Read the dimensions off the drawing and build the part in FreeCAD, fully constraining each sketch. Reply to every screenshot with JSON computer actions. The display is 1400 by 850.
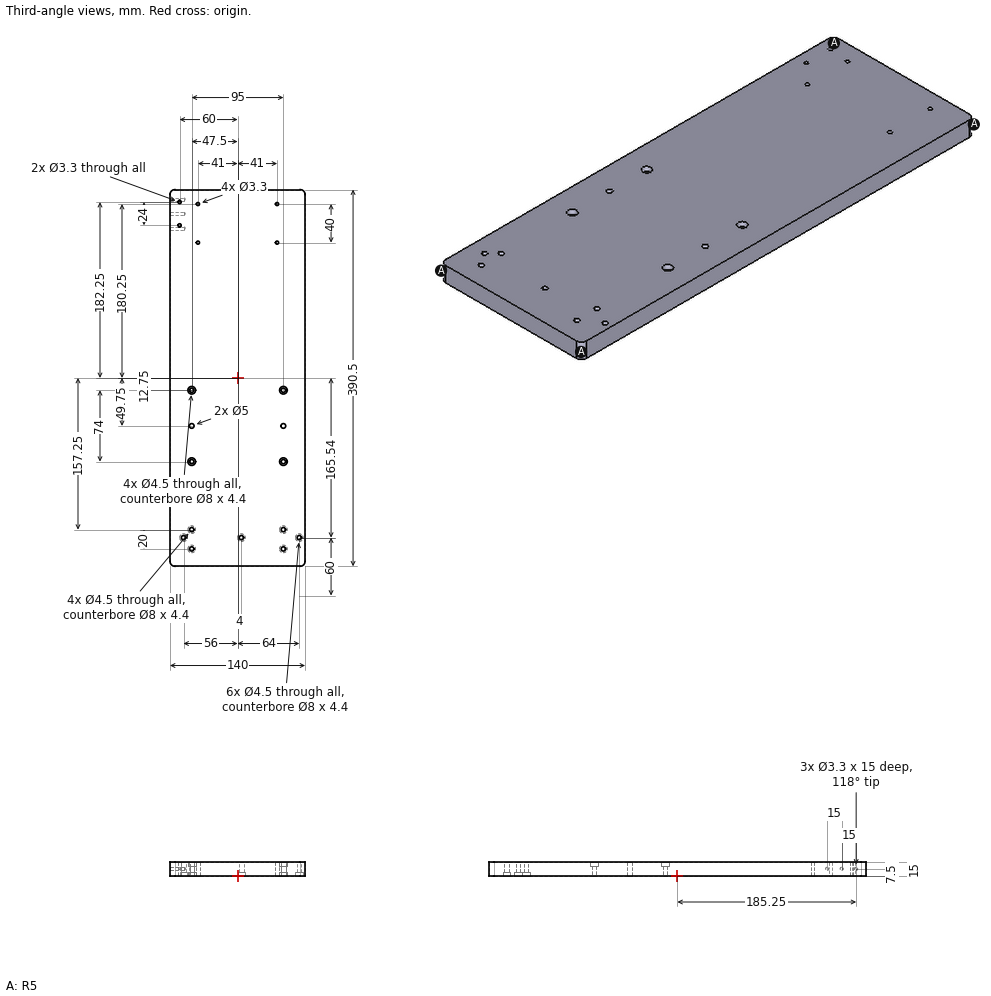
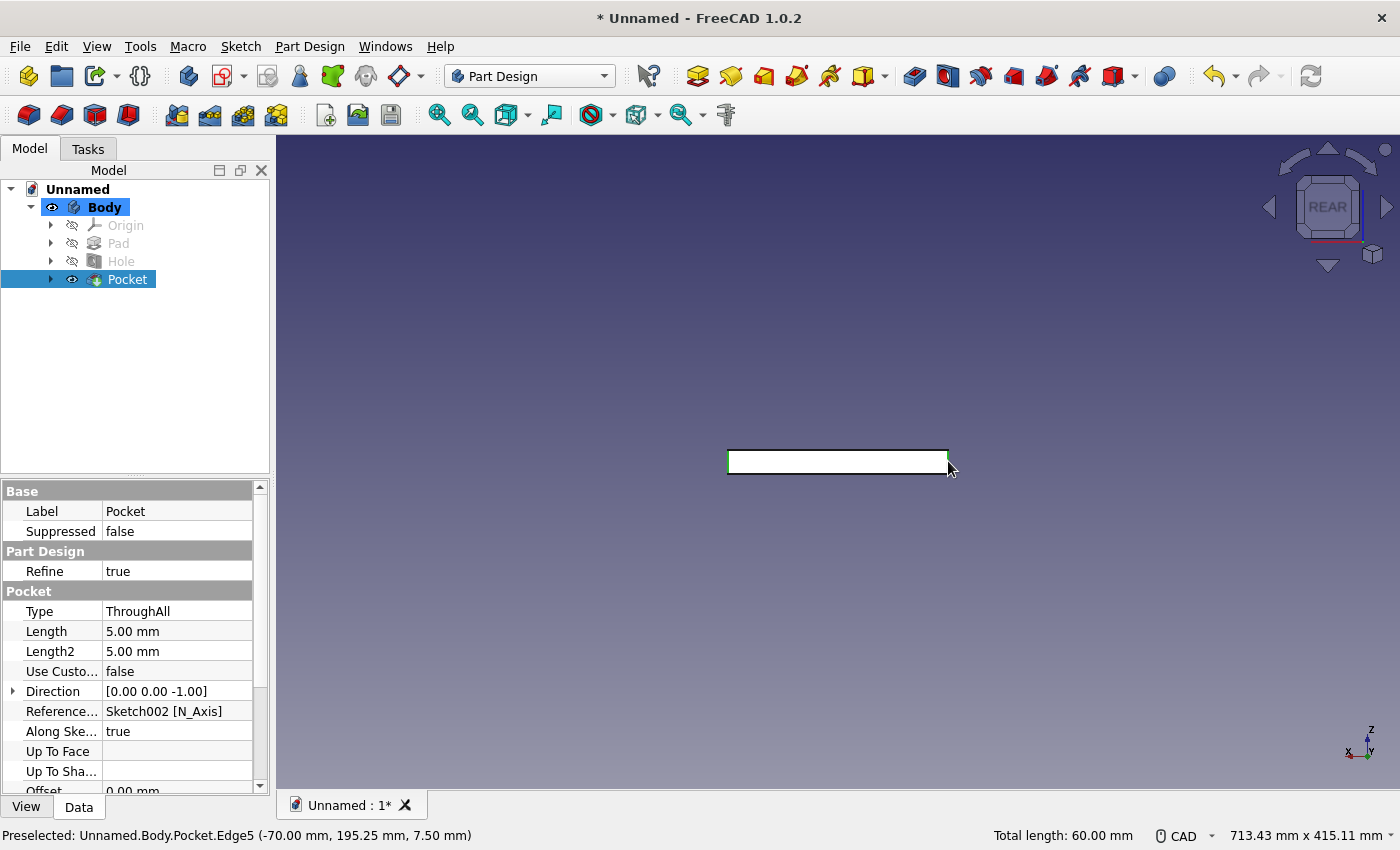
{"action": "left_click", "coordinate": [29, 116]}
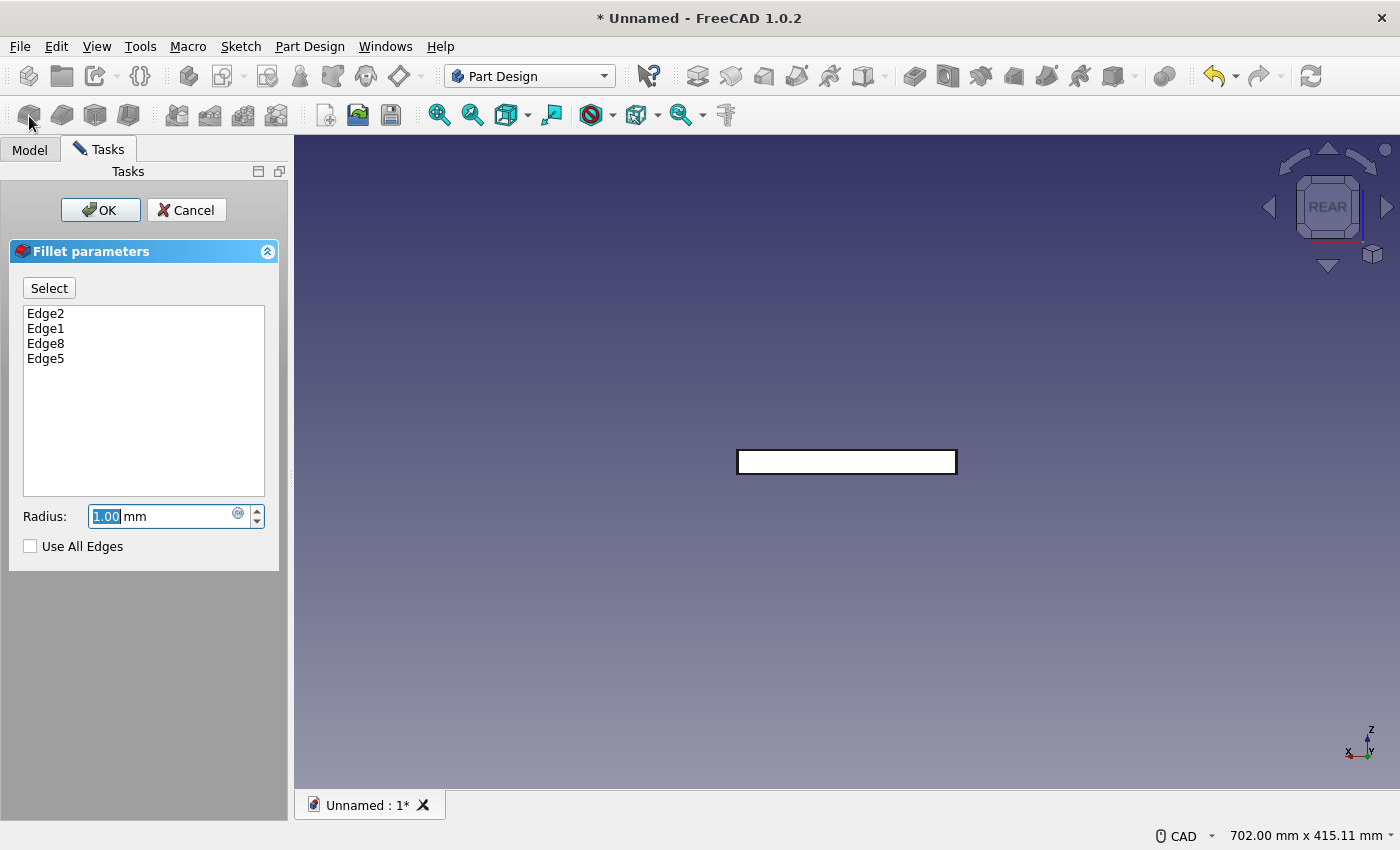
{"action": "type", "text": "5"}
{"action": "key", "text": "Tab"}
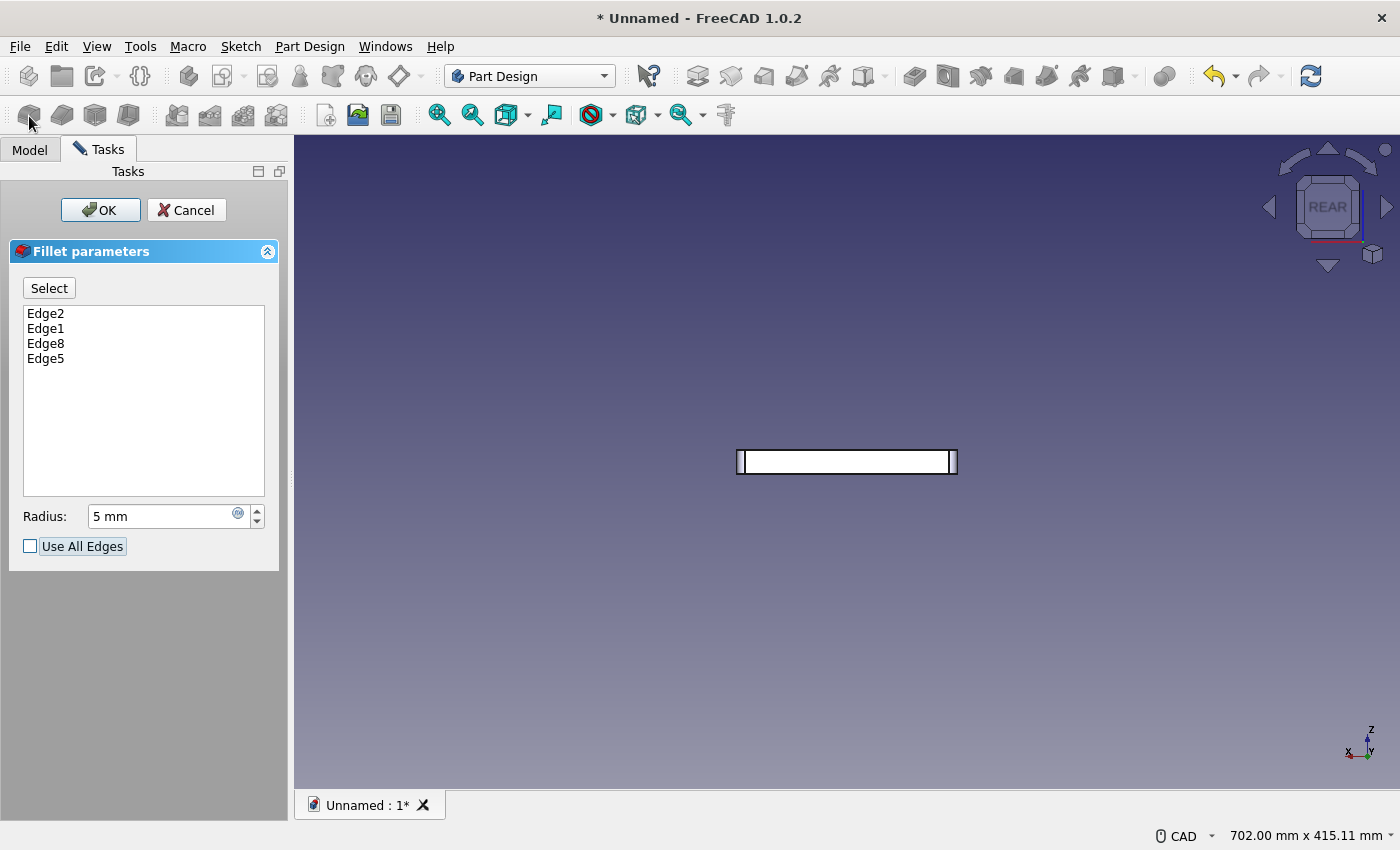
{"action": "left_click", "coordinate": [101, 210]}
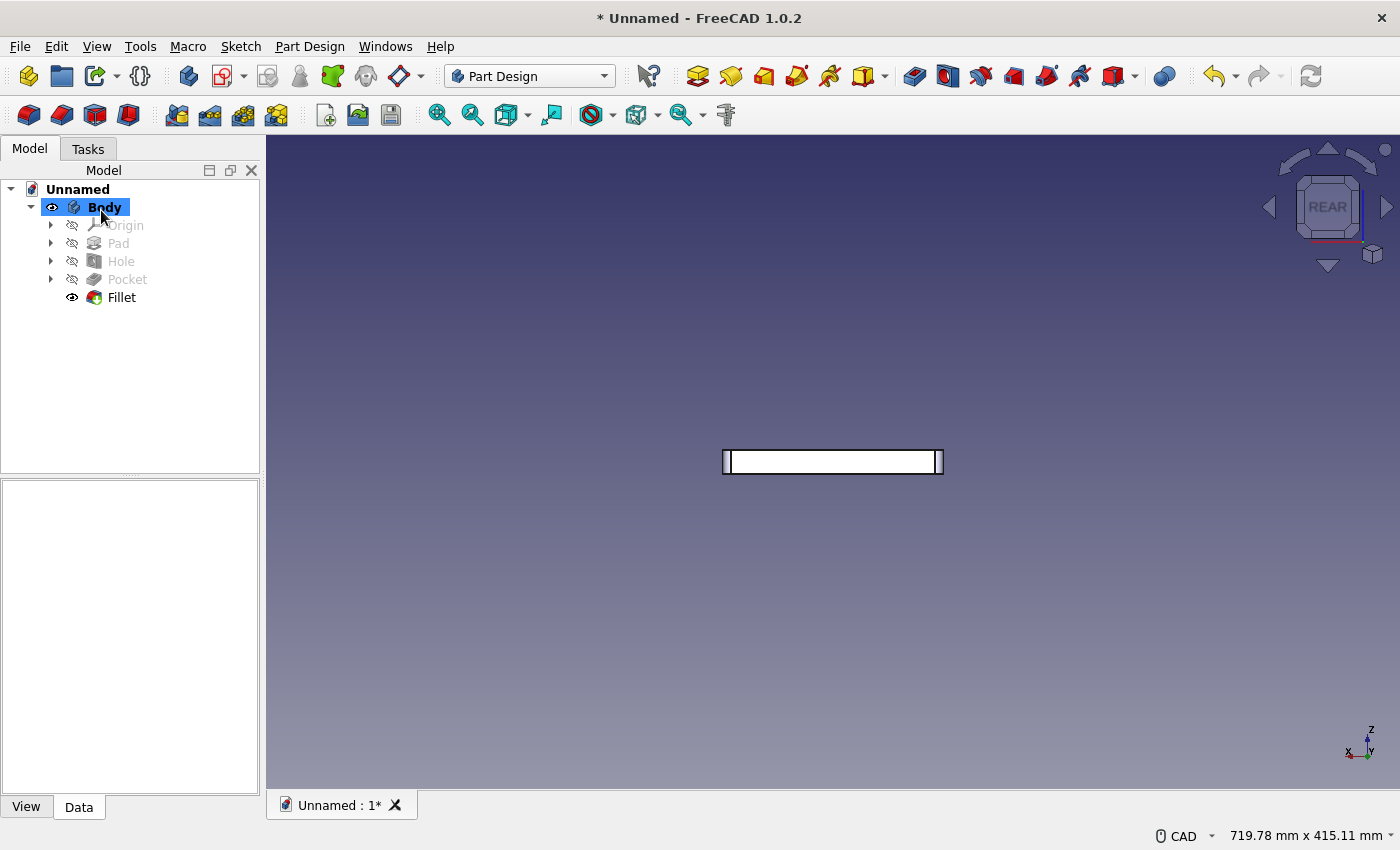
{"action": "left_click", "coordinate": [440, 116]}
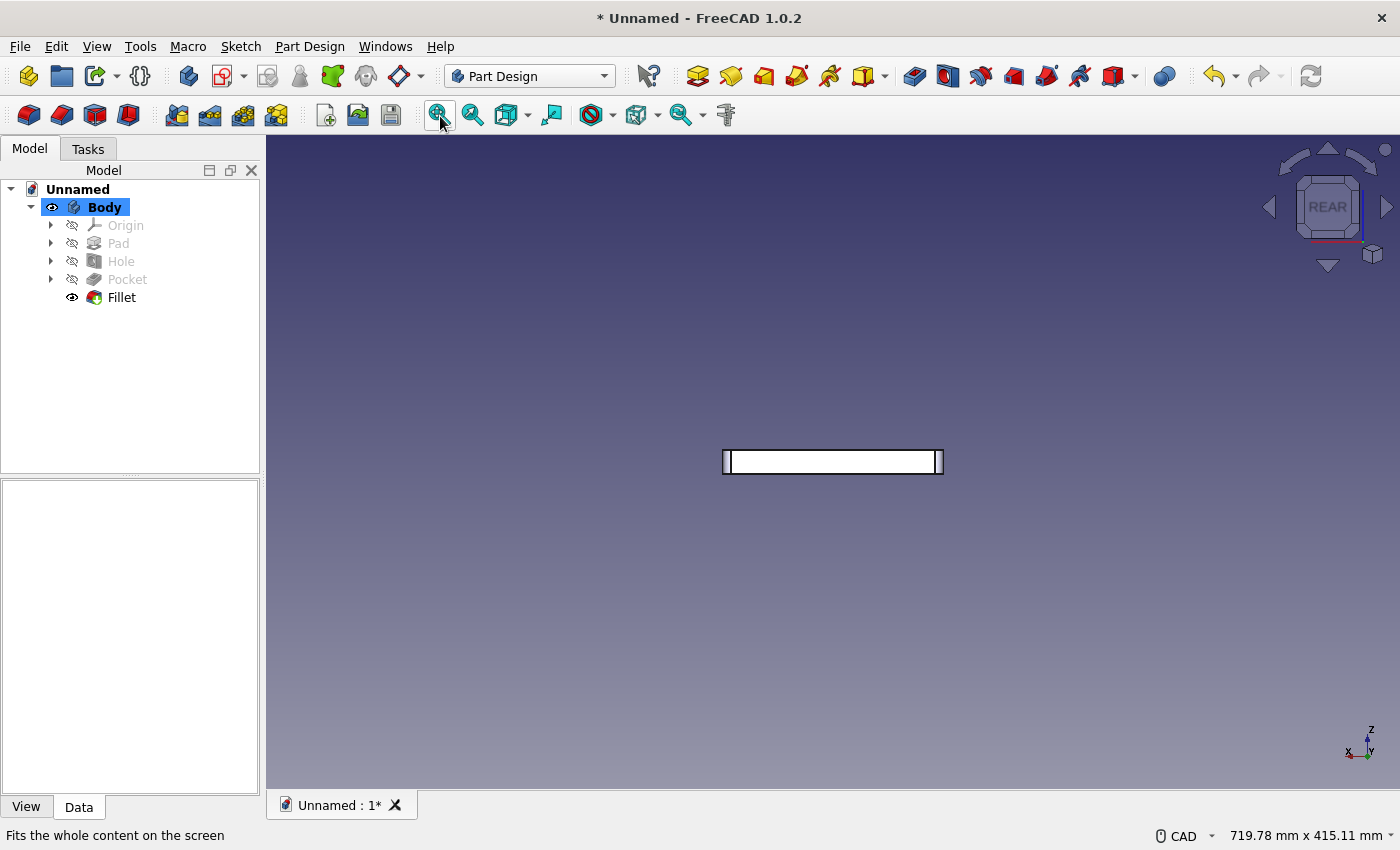
{"action": "key", "text": "0"}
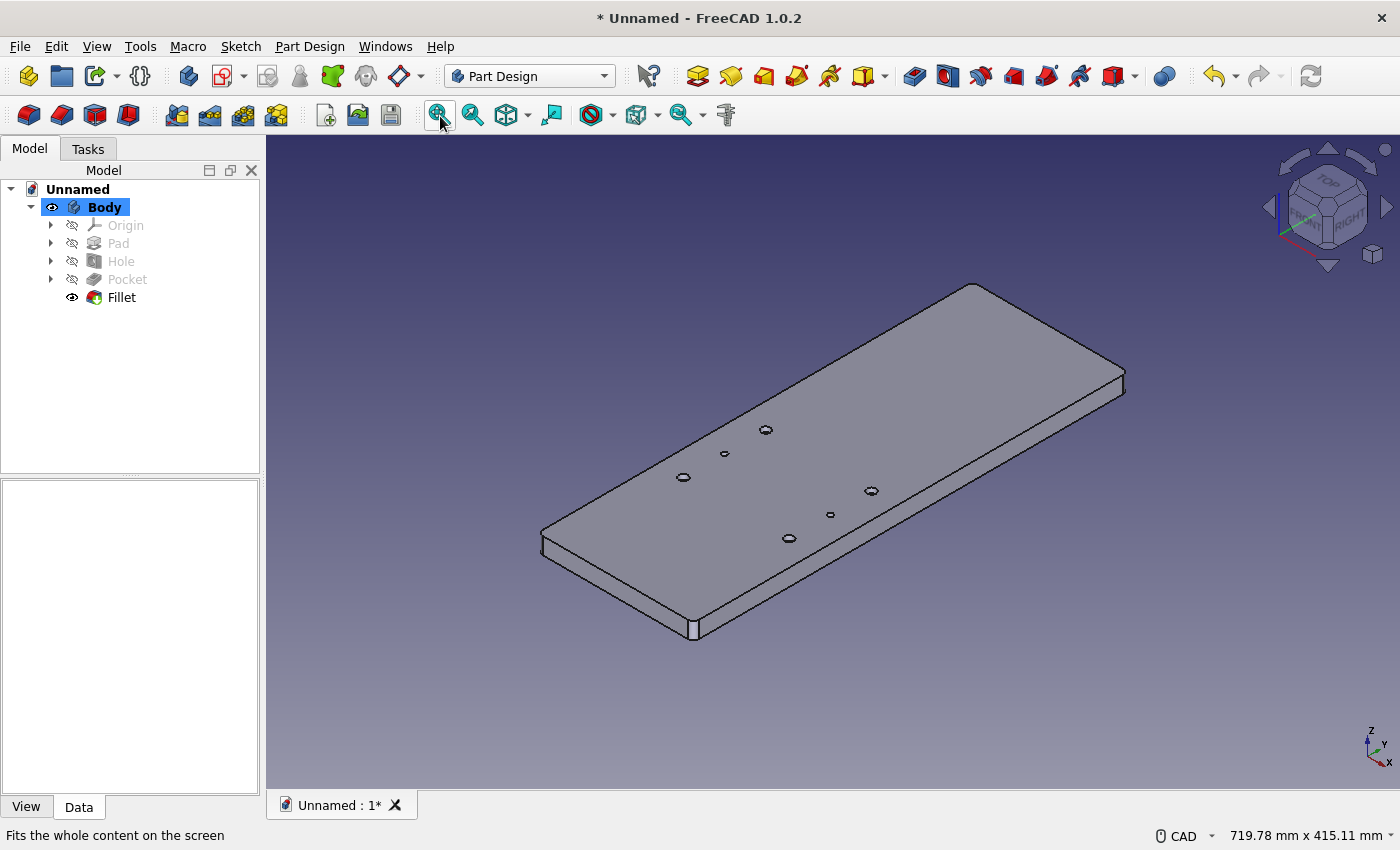
{"action": "left_click", "coordinate": [957, 380]}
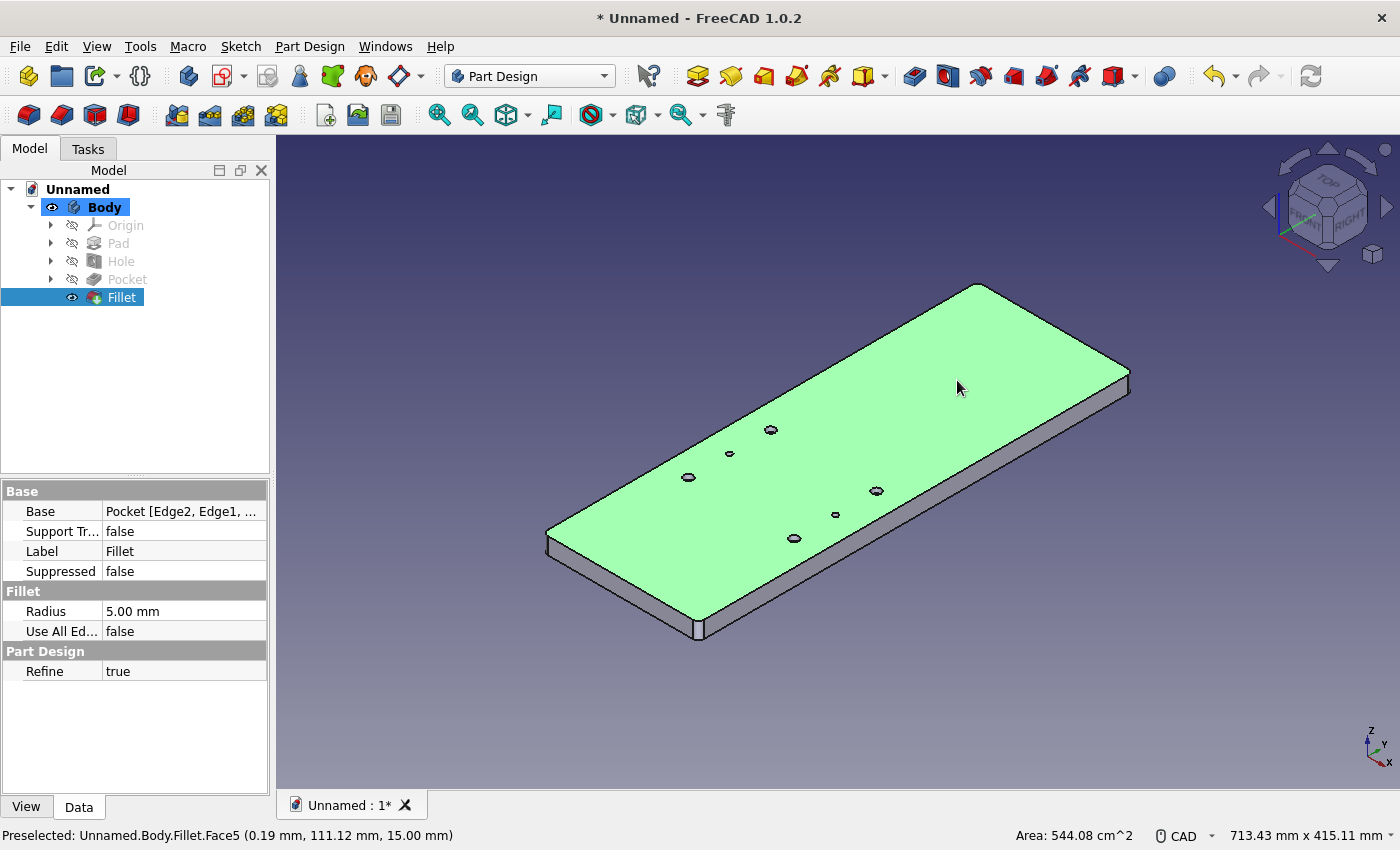
{"action": "left_click", "coordinate": [222, 76]}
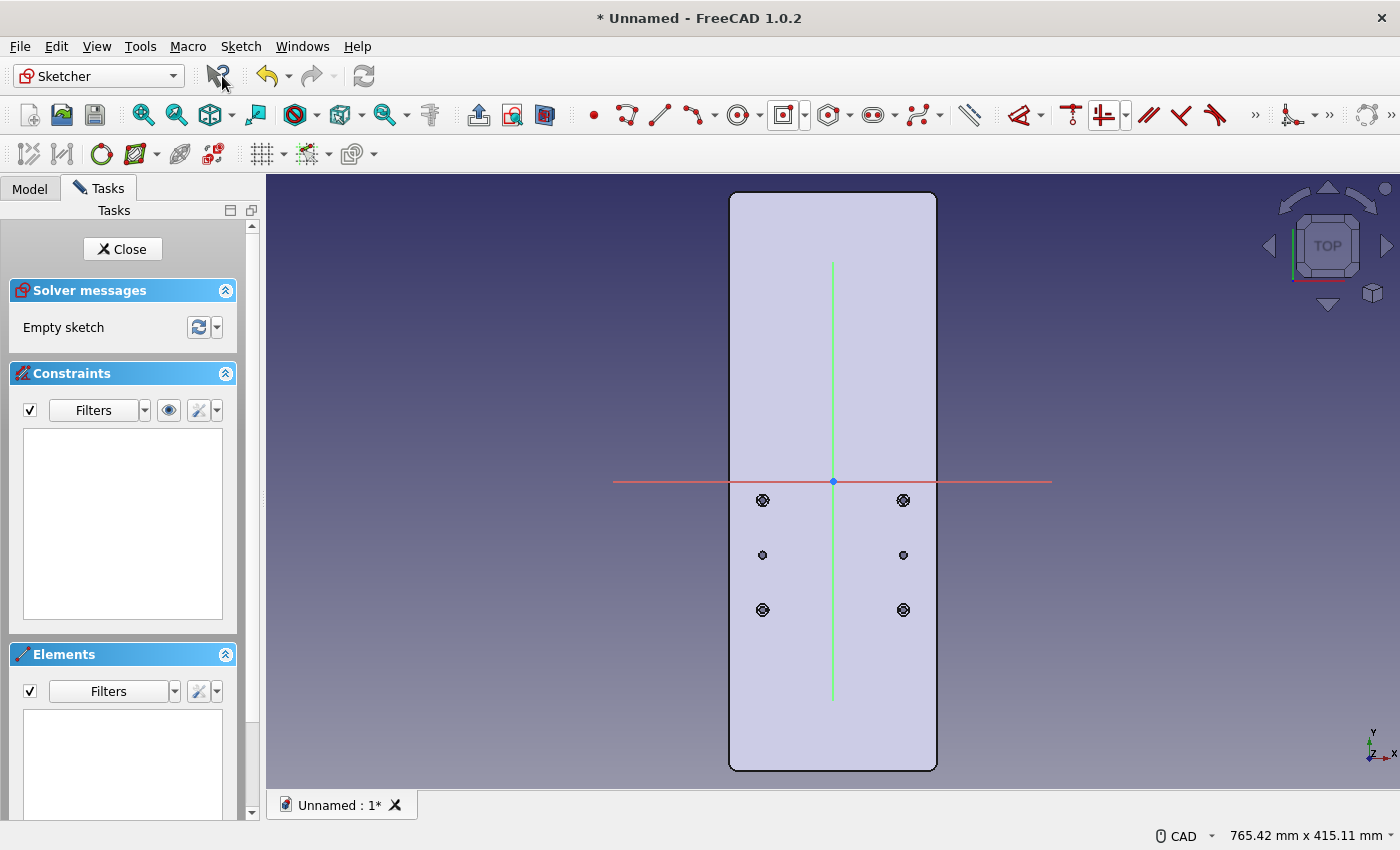
{"action": "scroll", "coordinate": [455, 761], "scroll_direction": "down", "scroll_amount": 1}